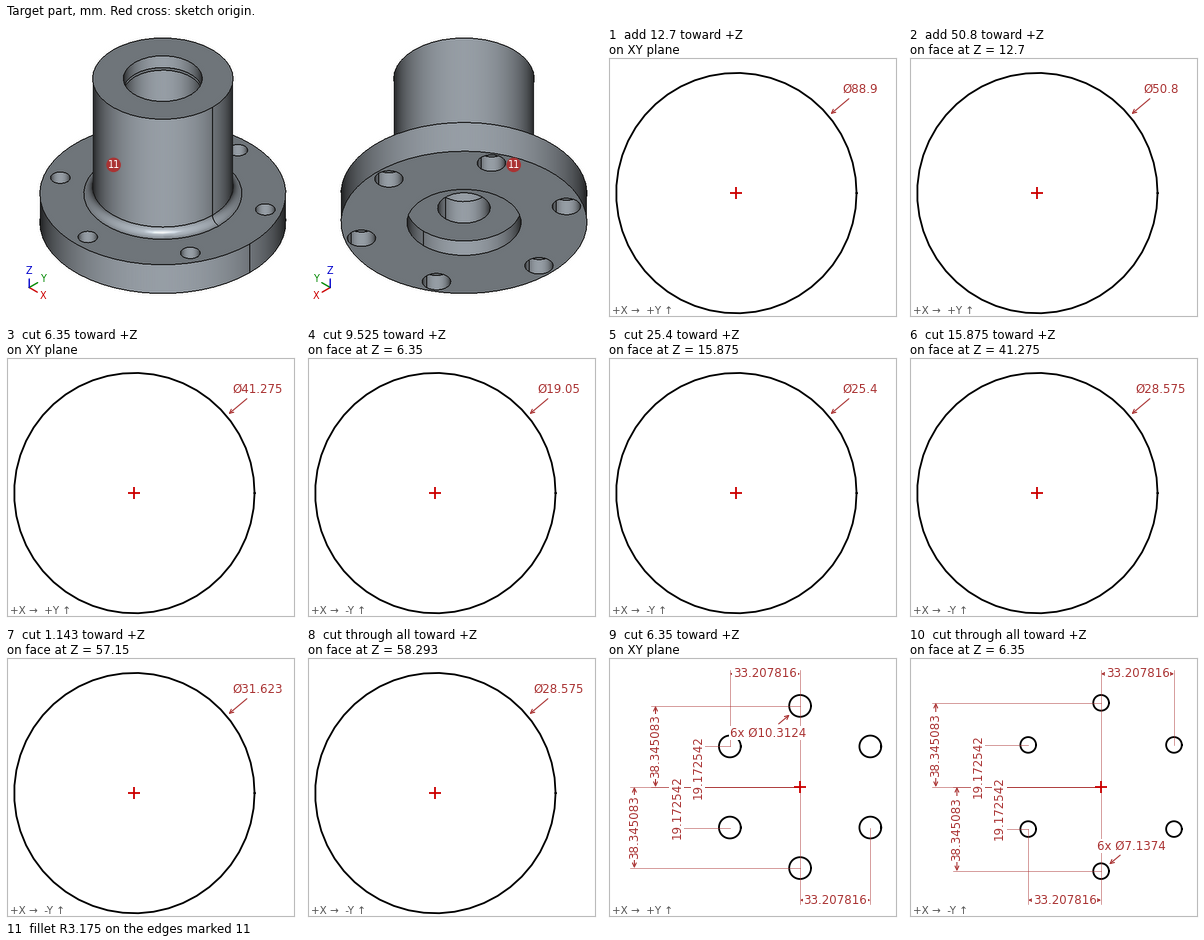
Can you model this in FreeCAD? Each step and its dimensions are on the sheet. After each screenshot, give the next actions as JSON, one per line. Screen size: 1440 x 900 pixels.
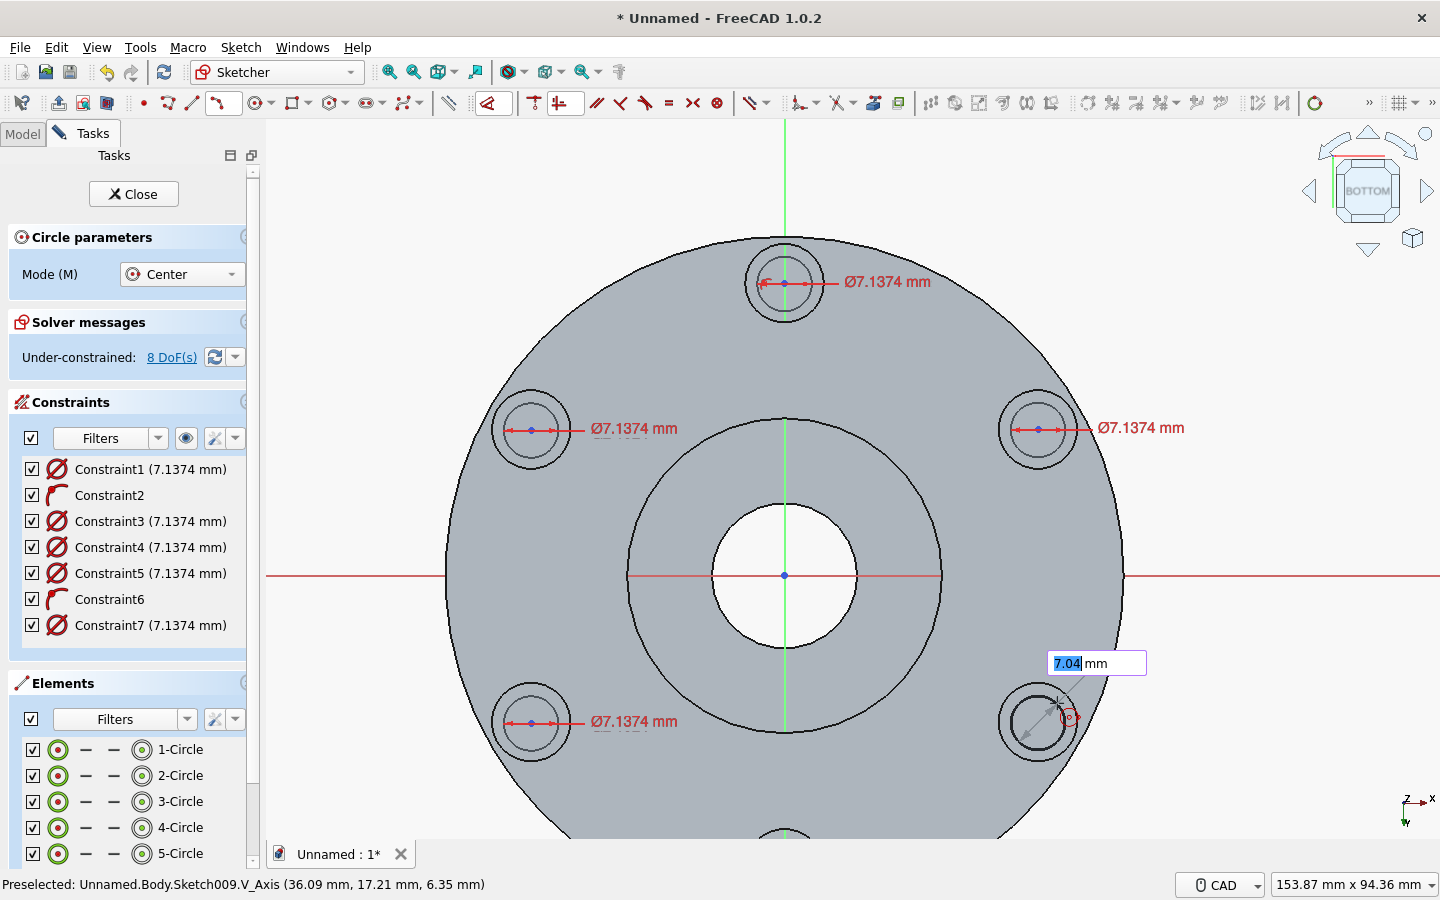
{"action": "type", "text": "7.1374"}
{"action": "key", "text": "Return"}
{"action": "key", "text": "Escape"}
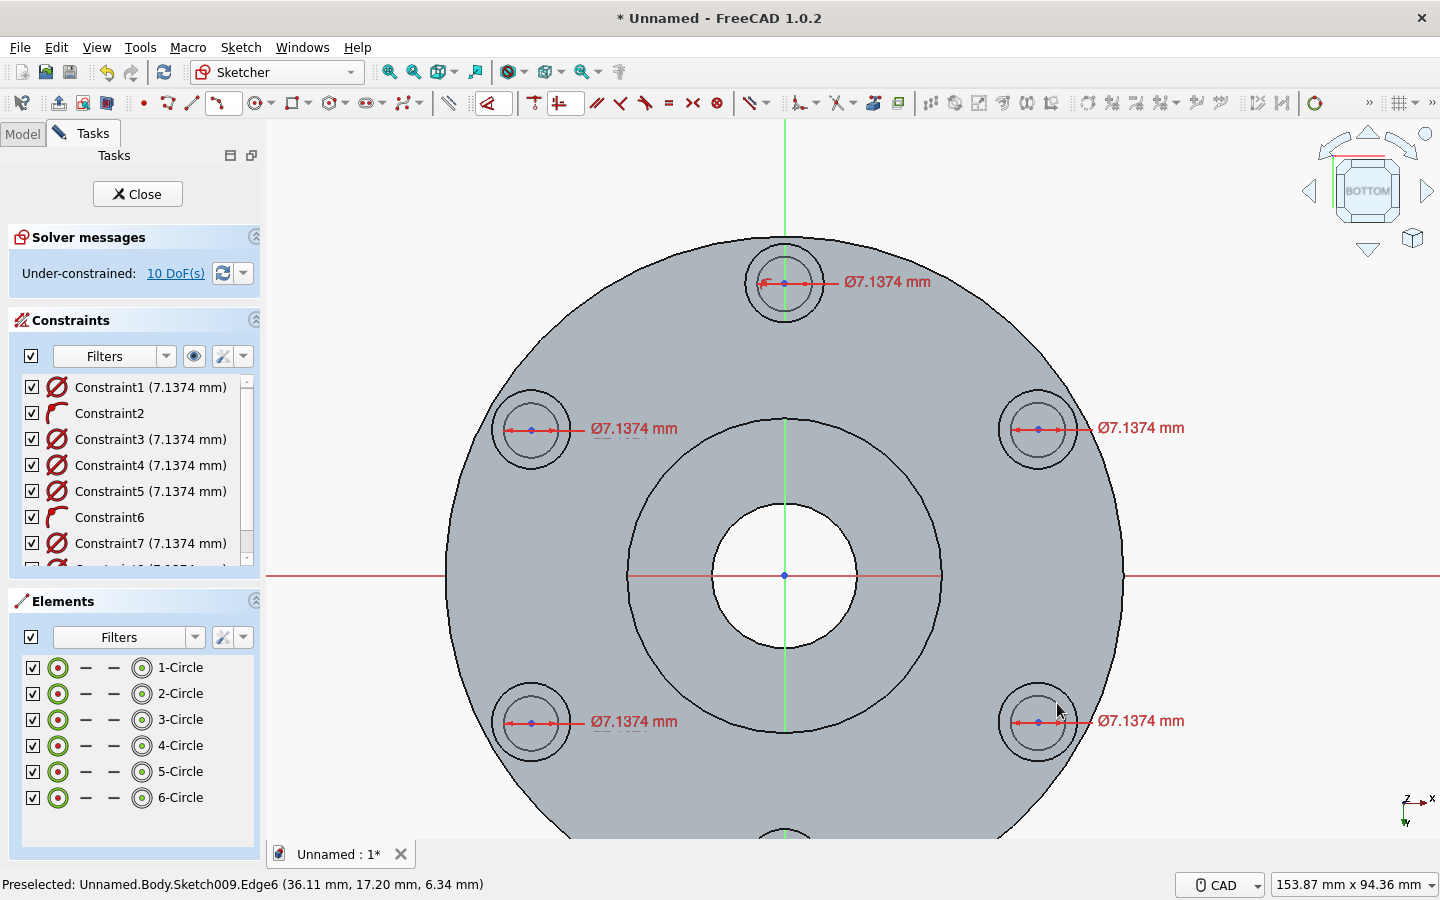
{"action": "left_click", "coordinate": [531, 724]}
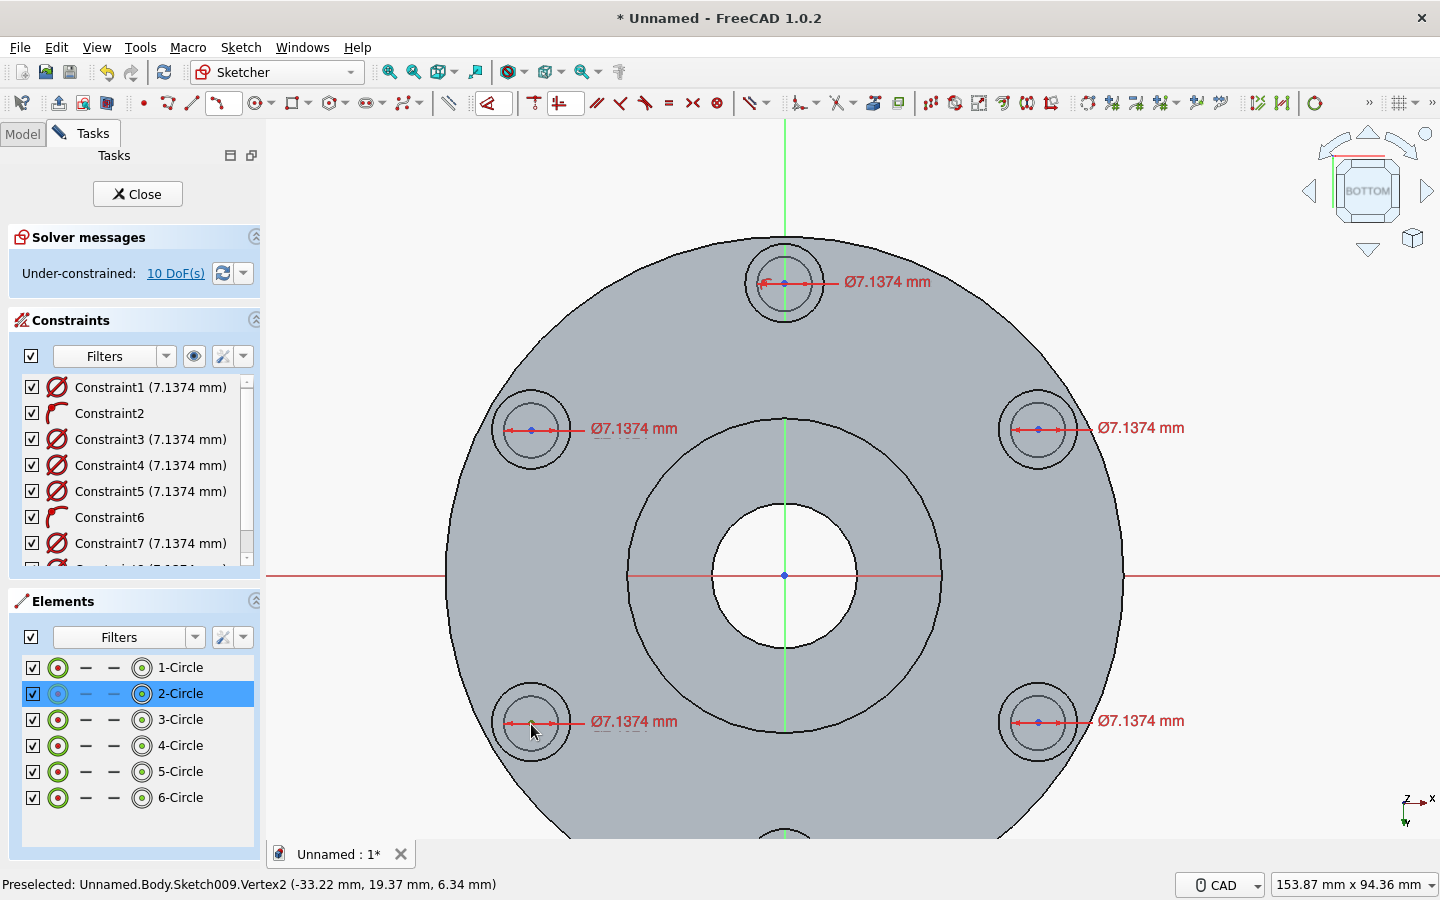
{"action": "left_click", "coordinate": [531, 431]}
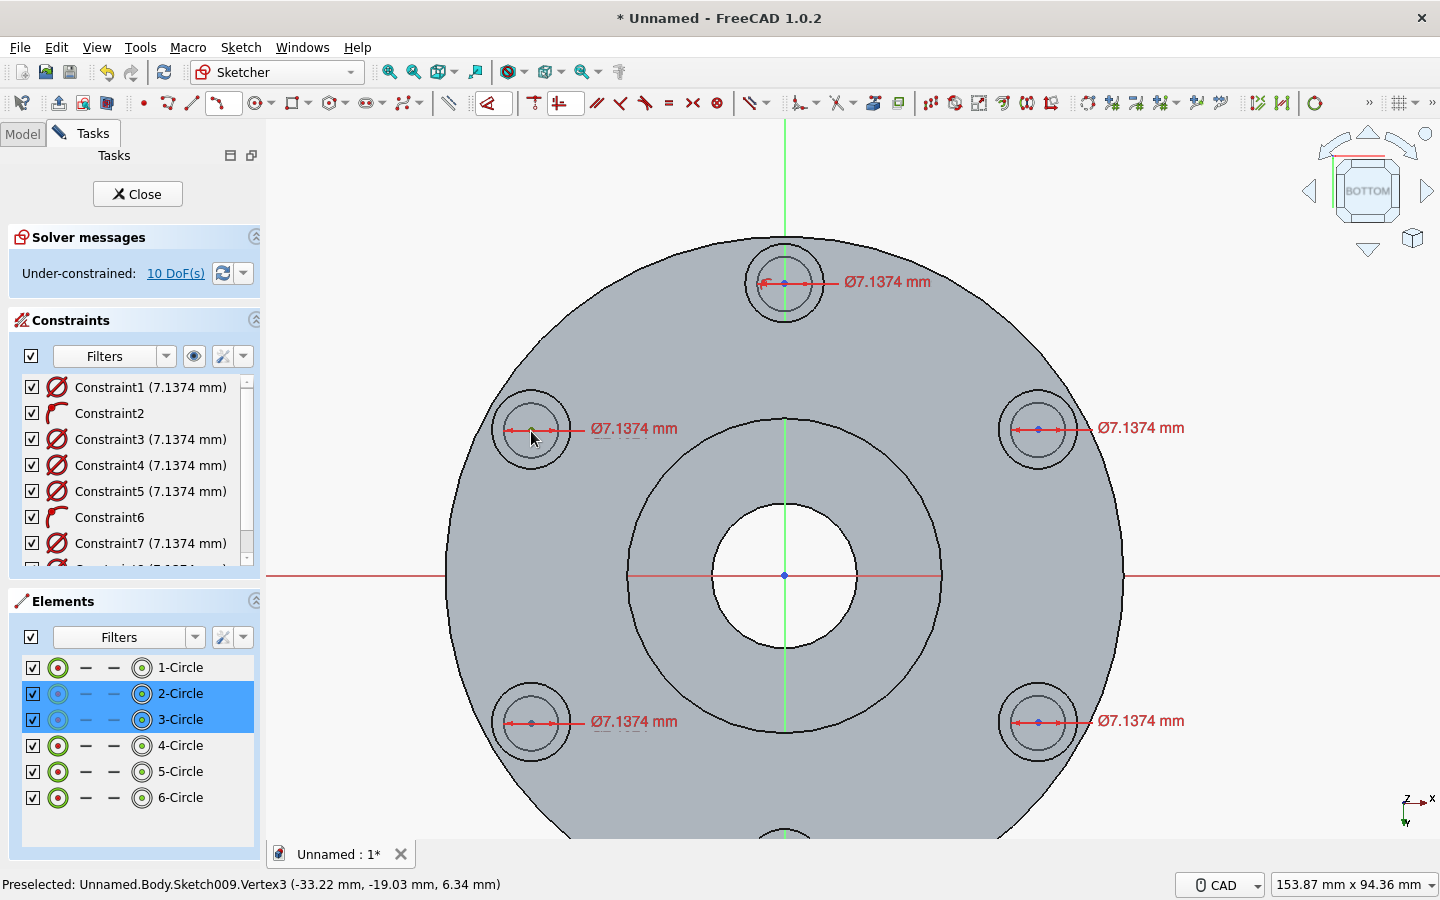
{"action": "key", "text": "v"}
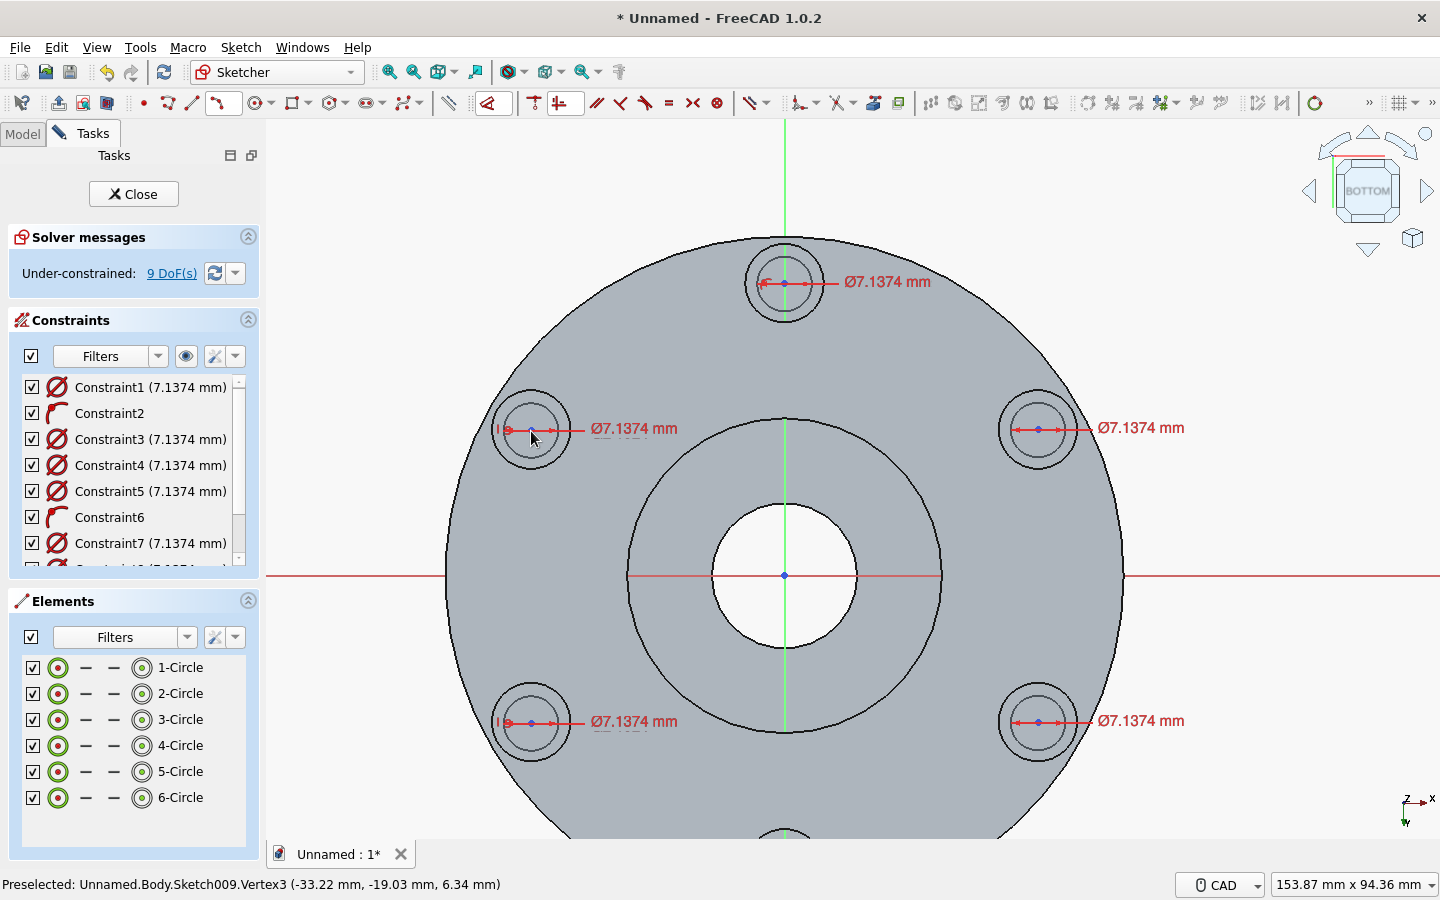
{"action": "left_click", "coordinate": [531, 431]}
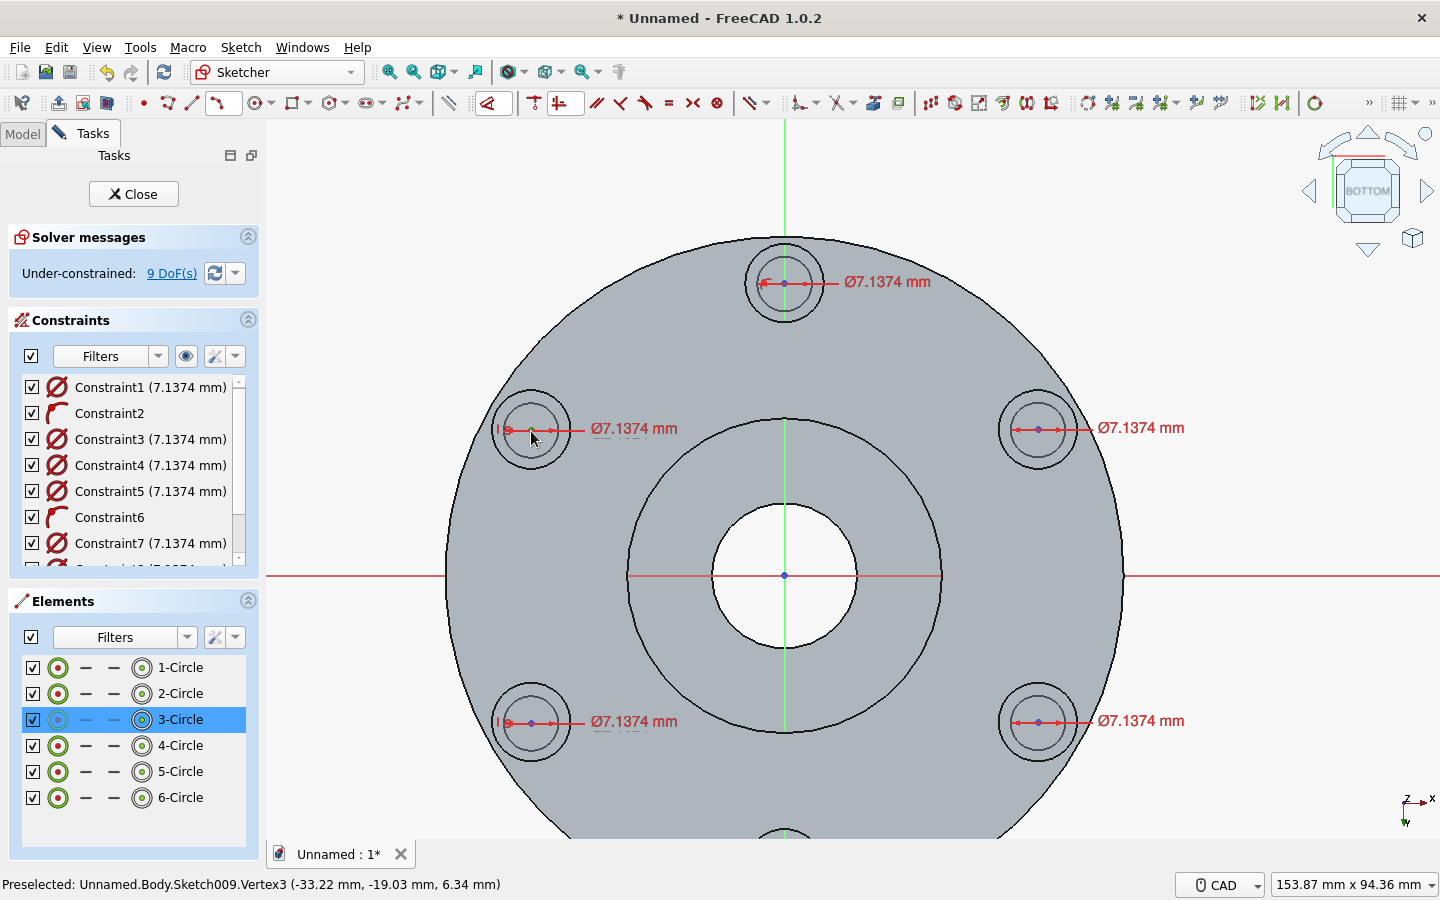
{"action": "left_click", "coordinate": [1038, 430]}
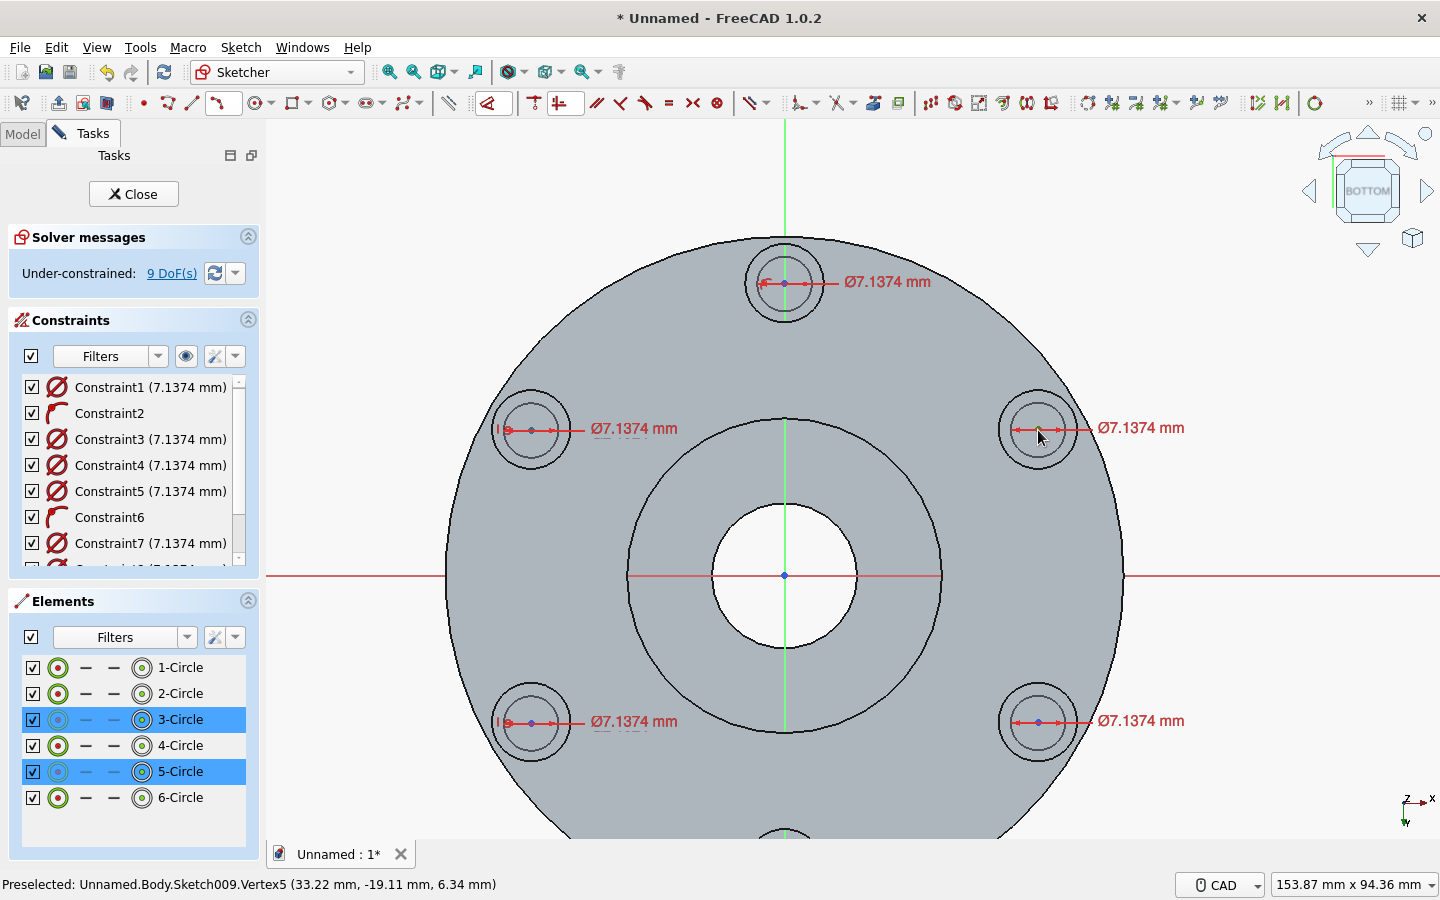
{"action": "key", "text": "h"}